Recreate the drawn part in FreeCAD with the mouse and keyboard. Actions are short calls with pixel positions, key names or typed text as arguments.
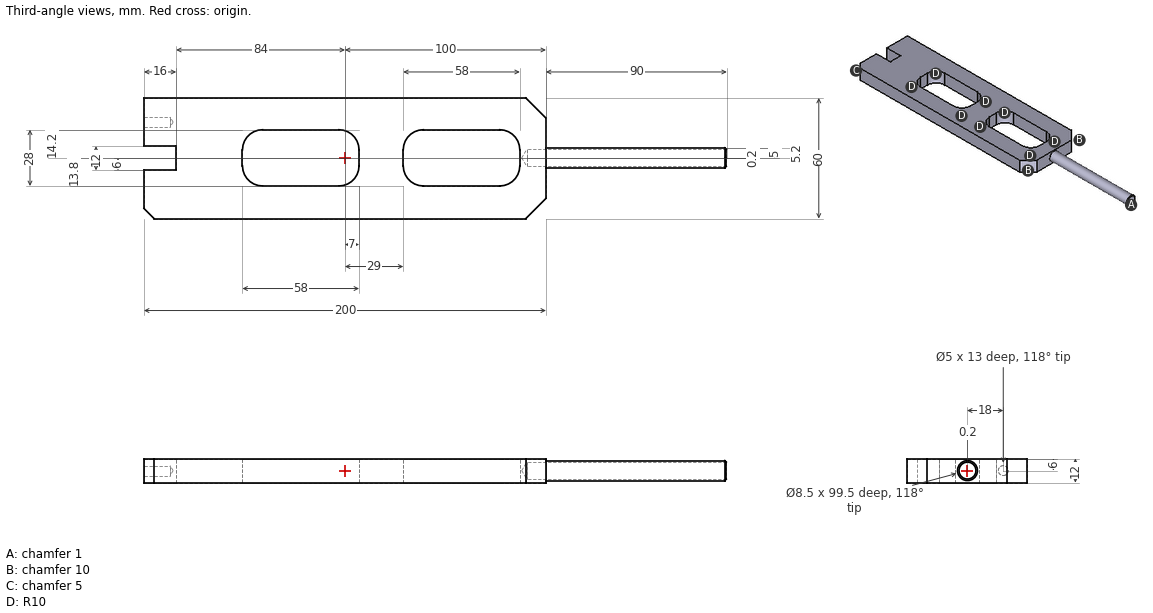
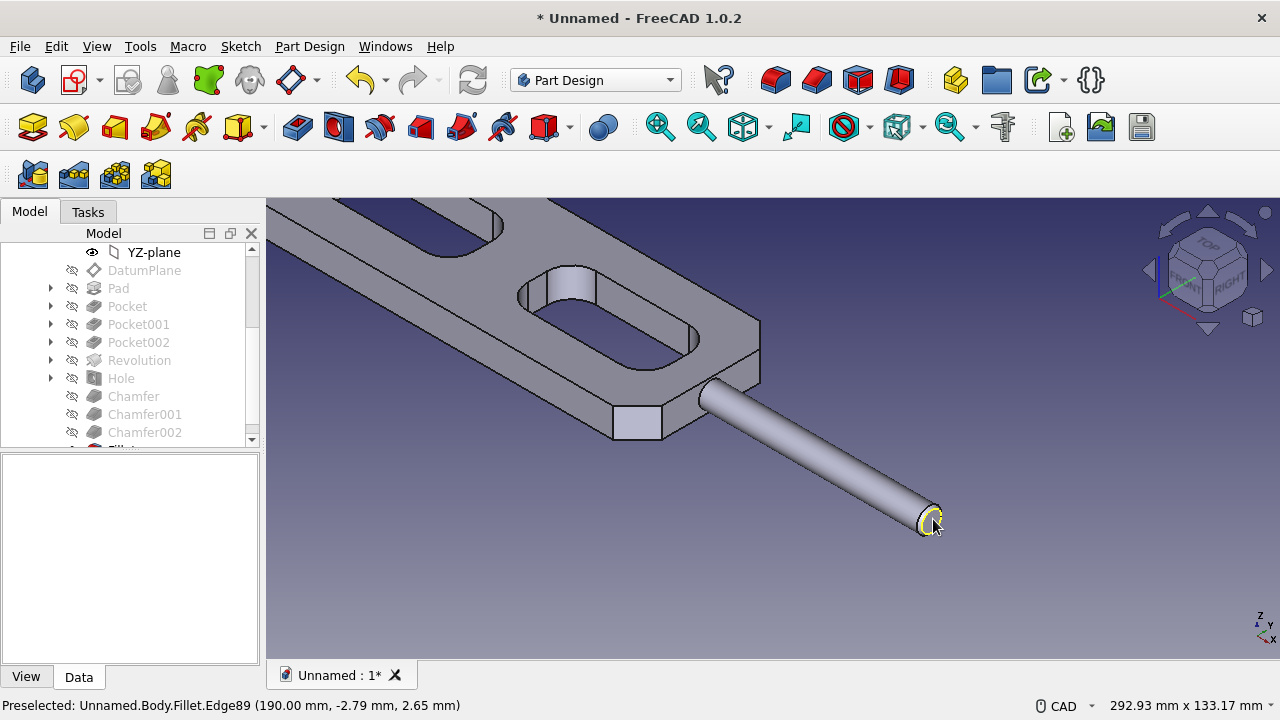
click(932, 524)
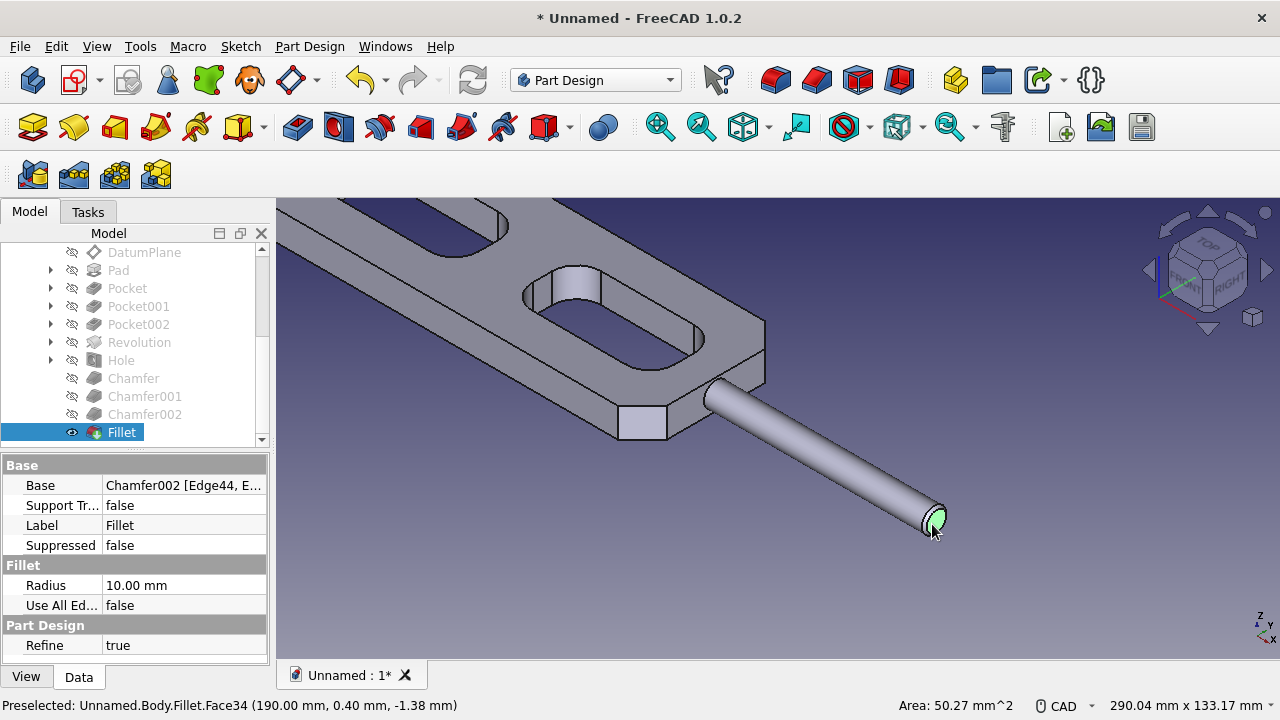
click(74, 80)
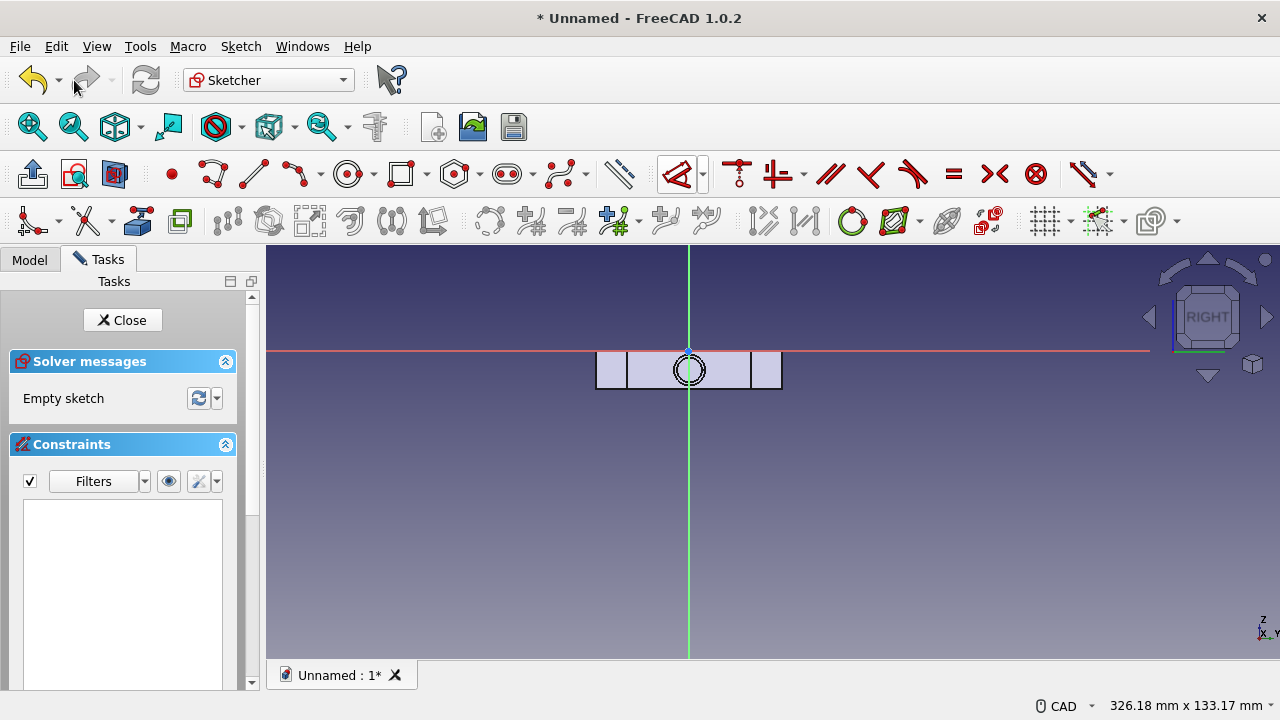
scroll(687, 354, up, 10)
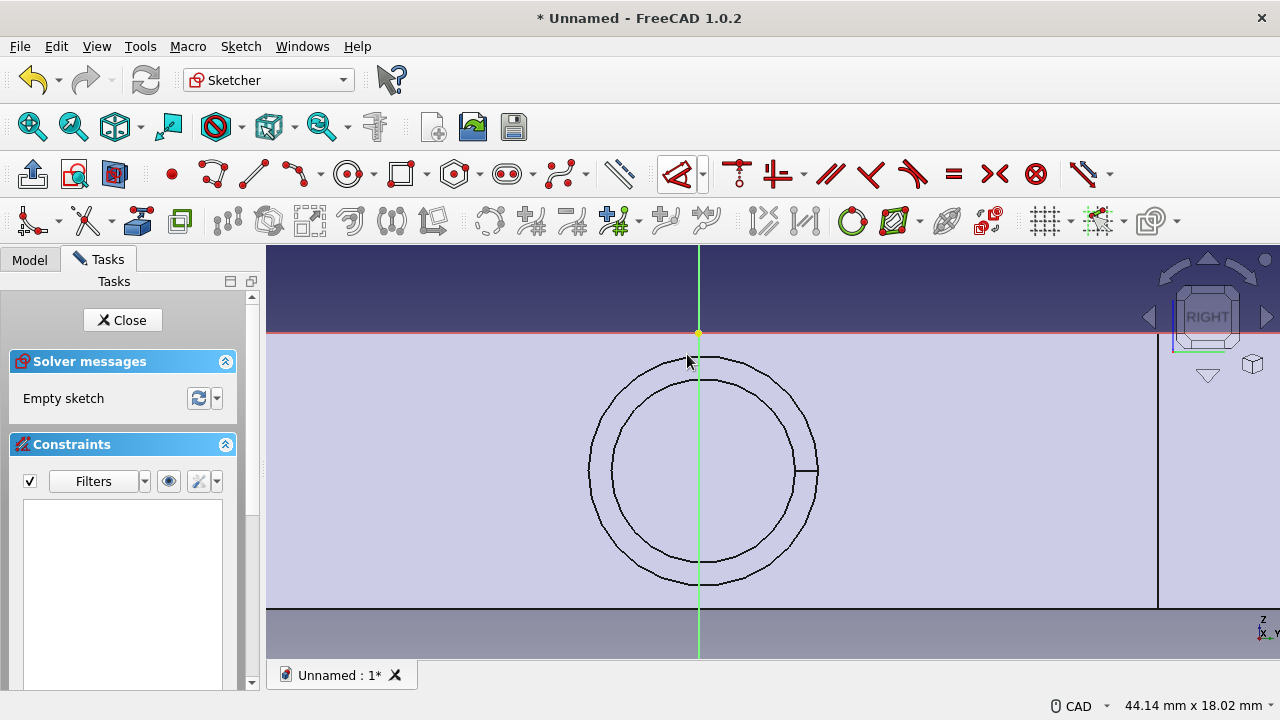
key(g)
key(c)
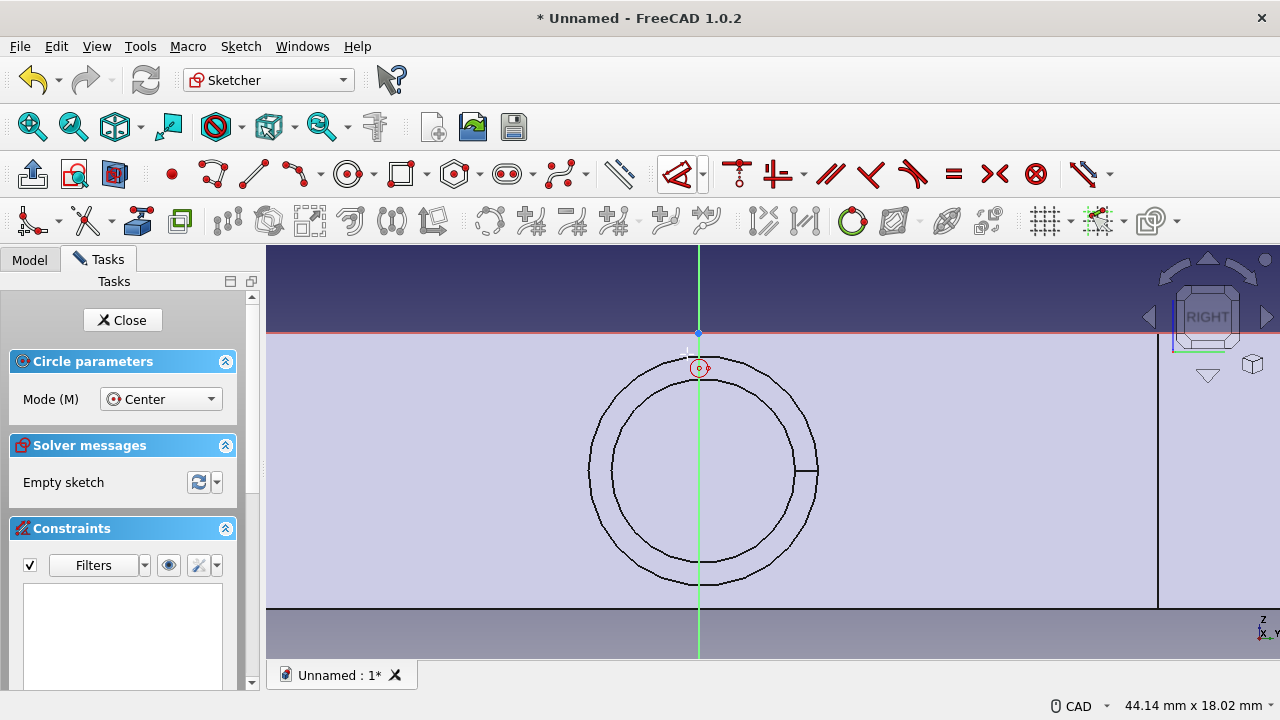
scroll(703, 471, up, 7)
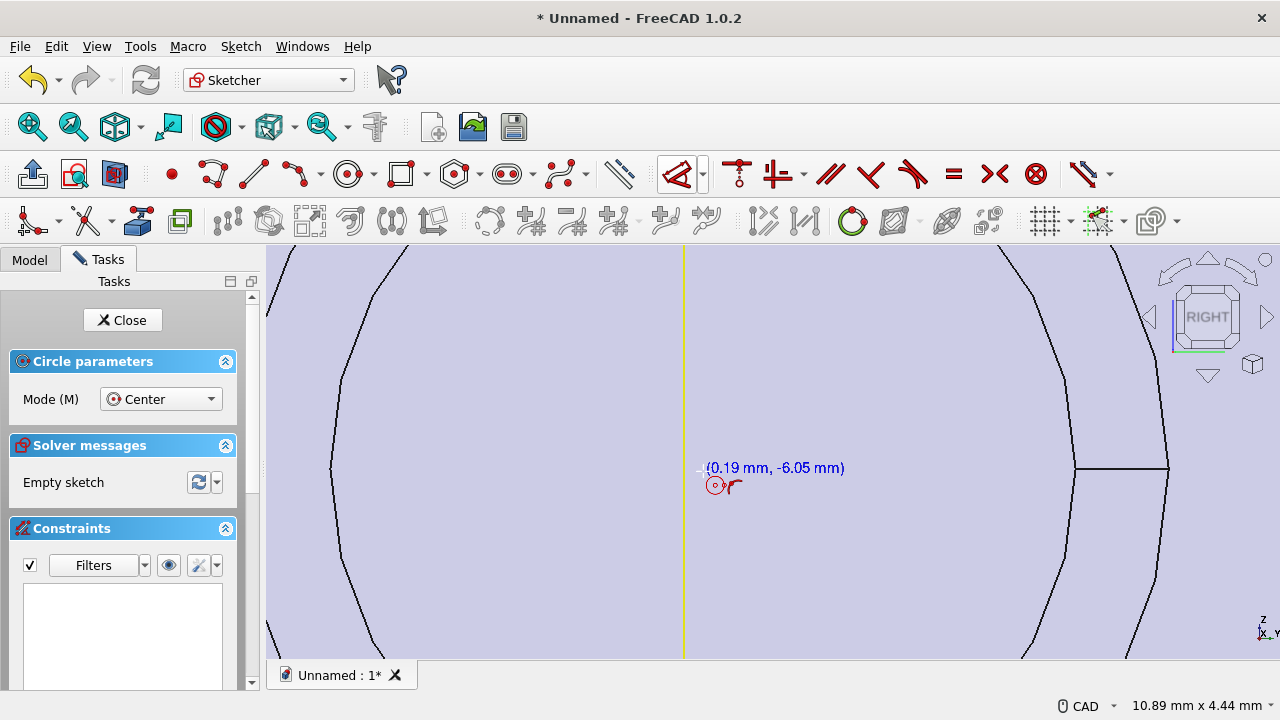
click(703, 469)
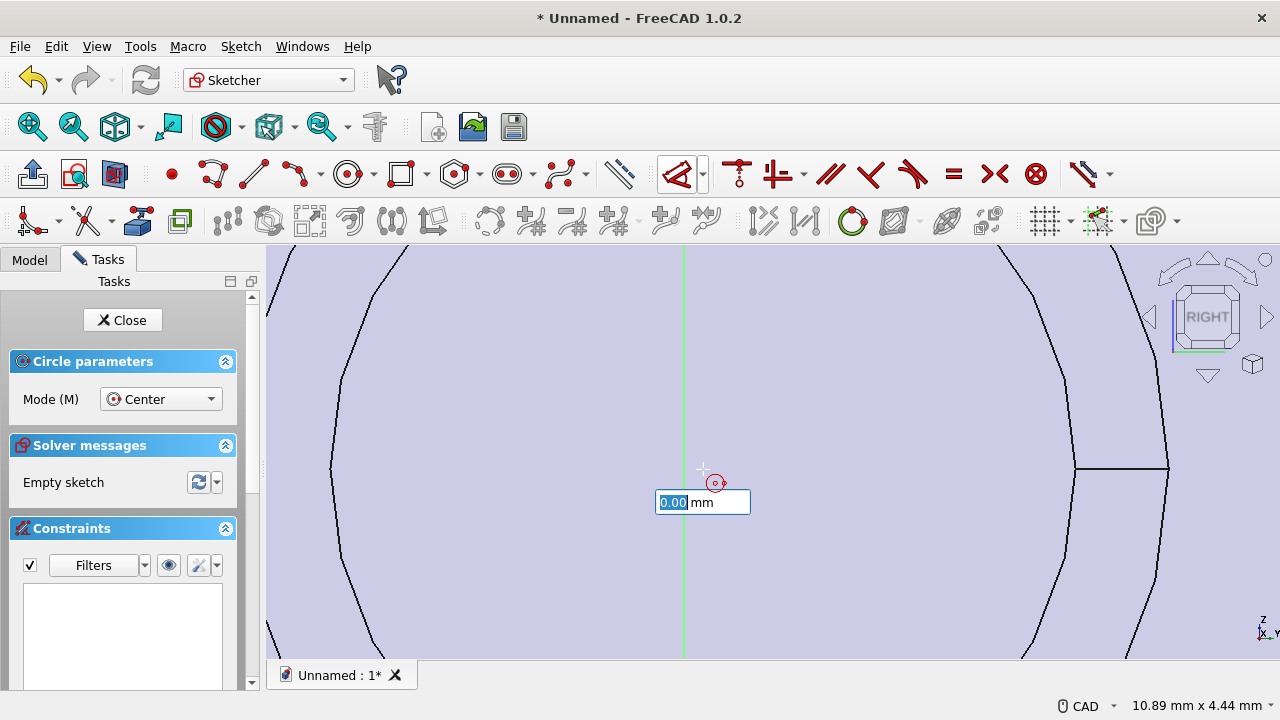
scroll(705, 473, down, 7)
move(774, 403)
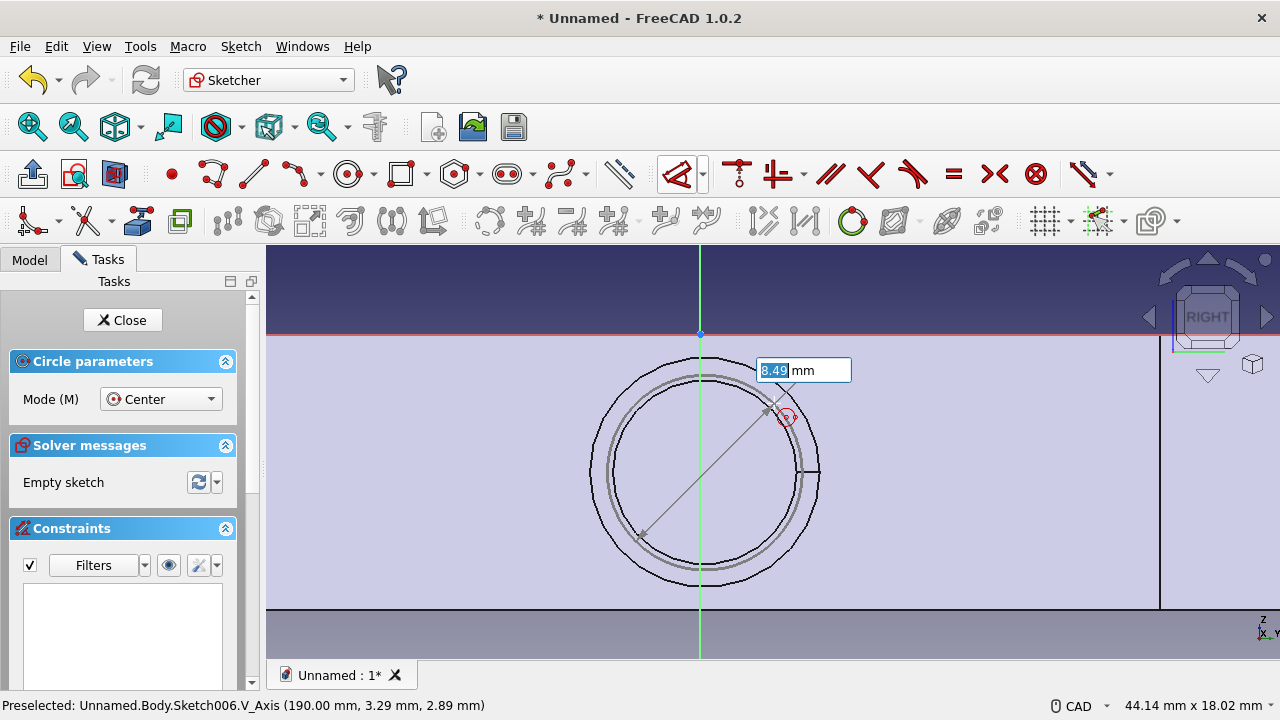
text(8.5)
key(Return)
key(Escape)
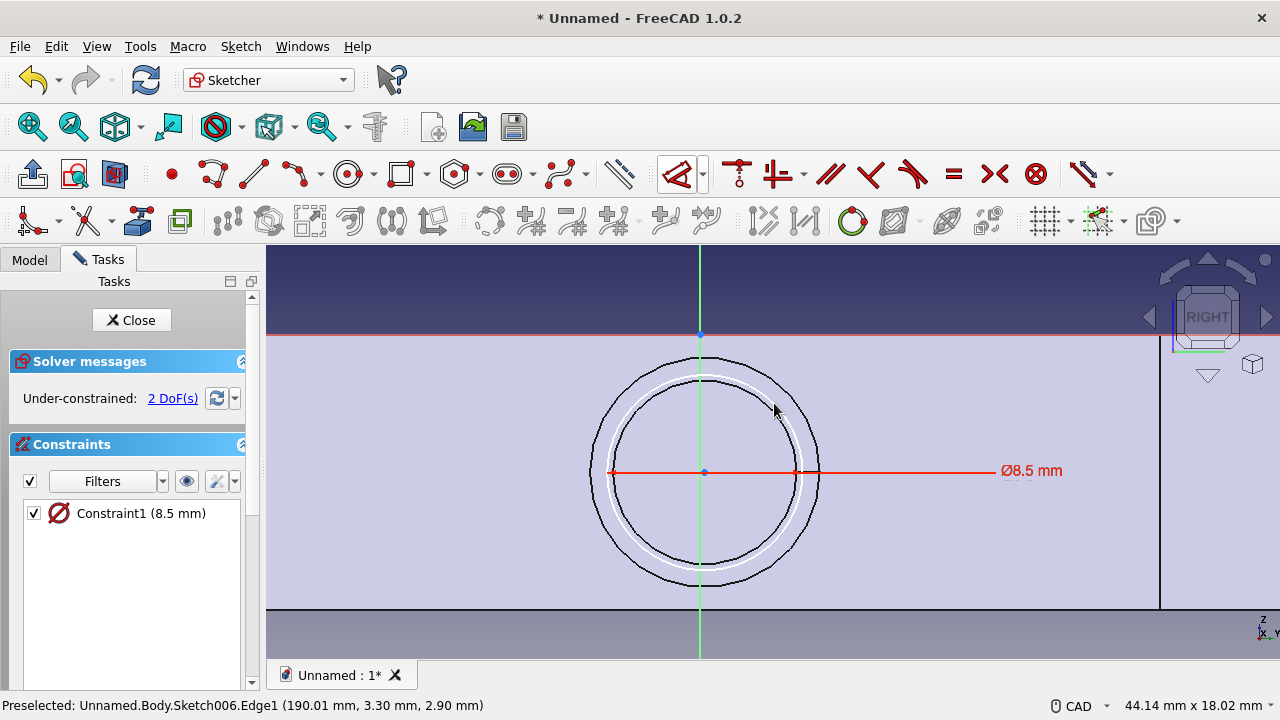
click(705, 473)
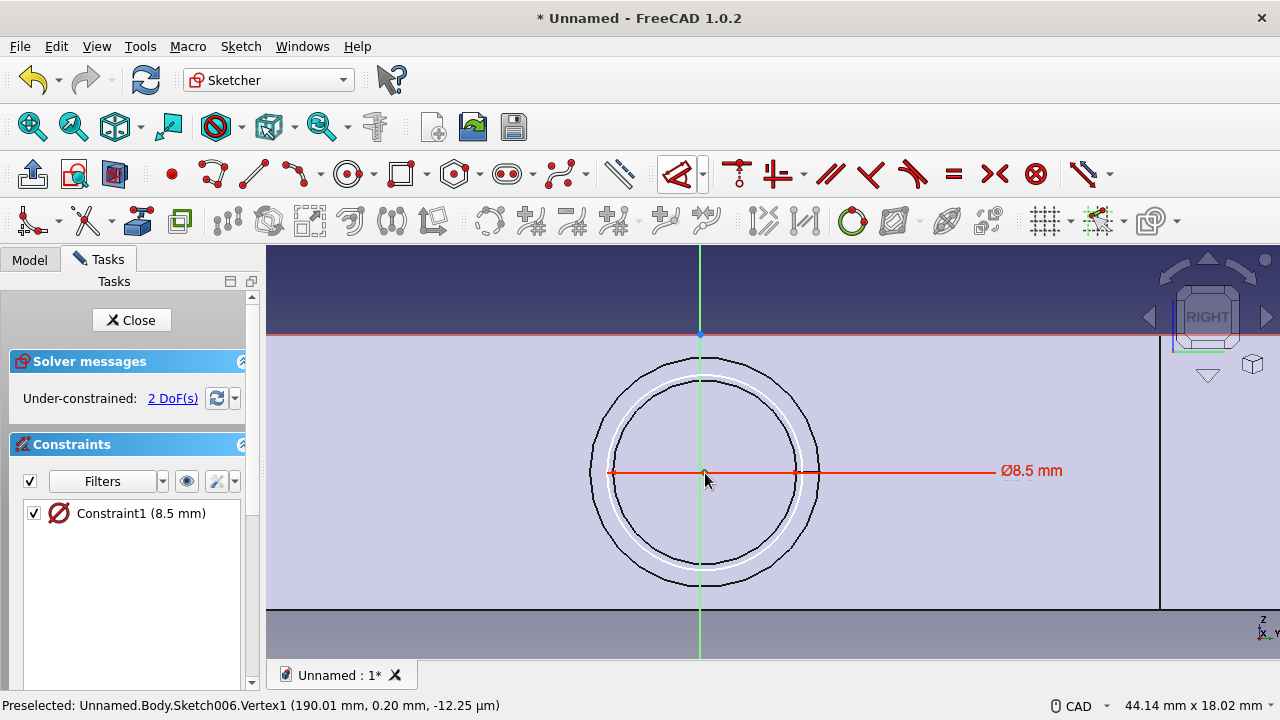
key(i)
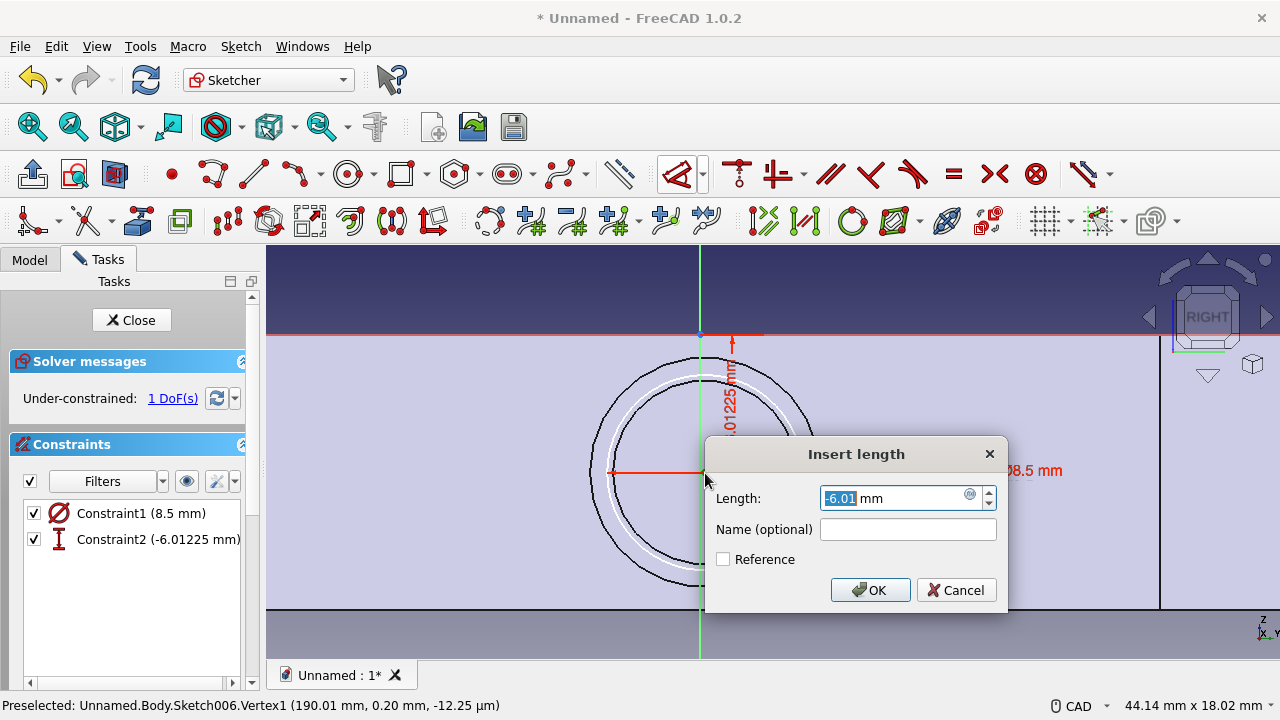
text(-6)
key(Return)